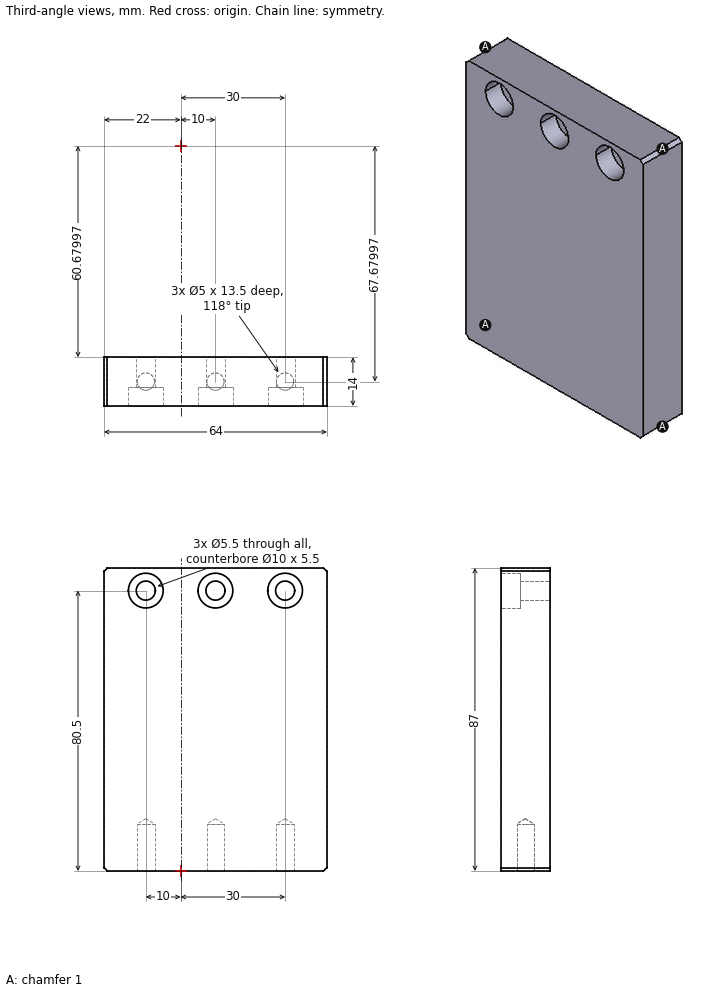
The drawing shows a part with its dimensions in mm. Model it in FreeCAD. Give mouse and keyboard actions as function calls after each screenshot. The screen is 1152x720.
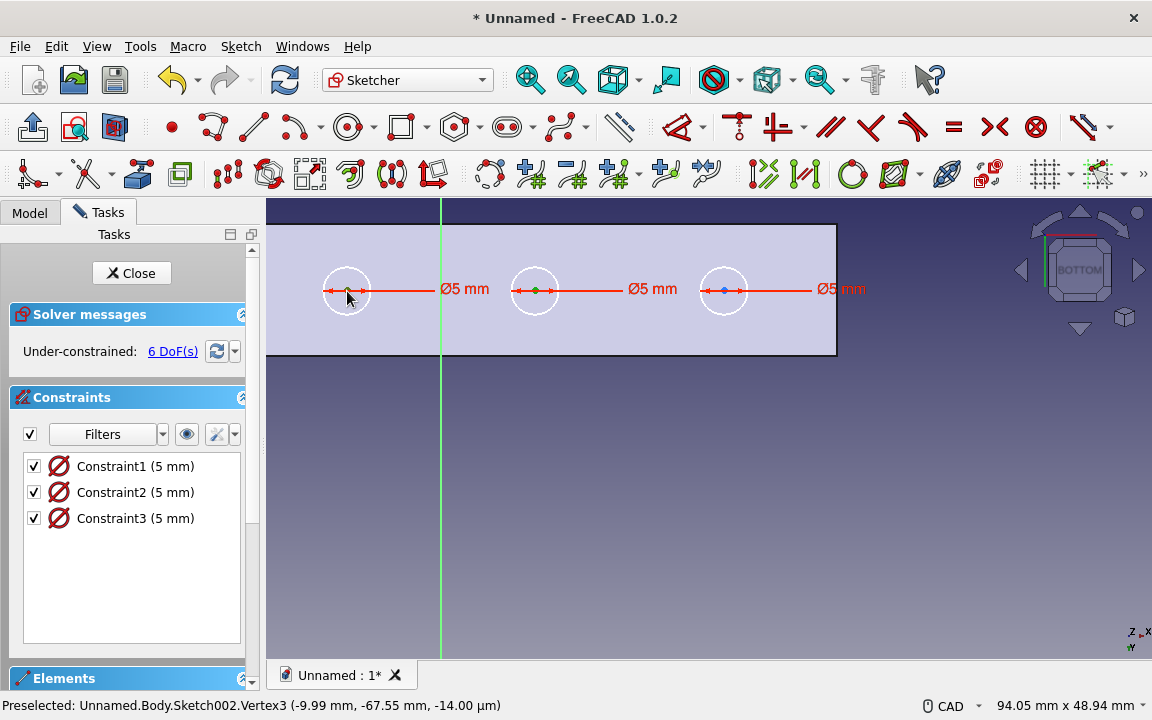
click(441, 602)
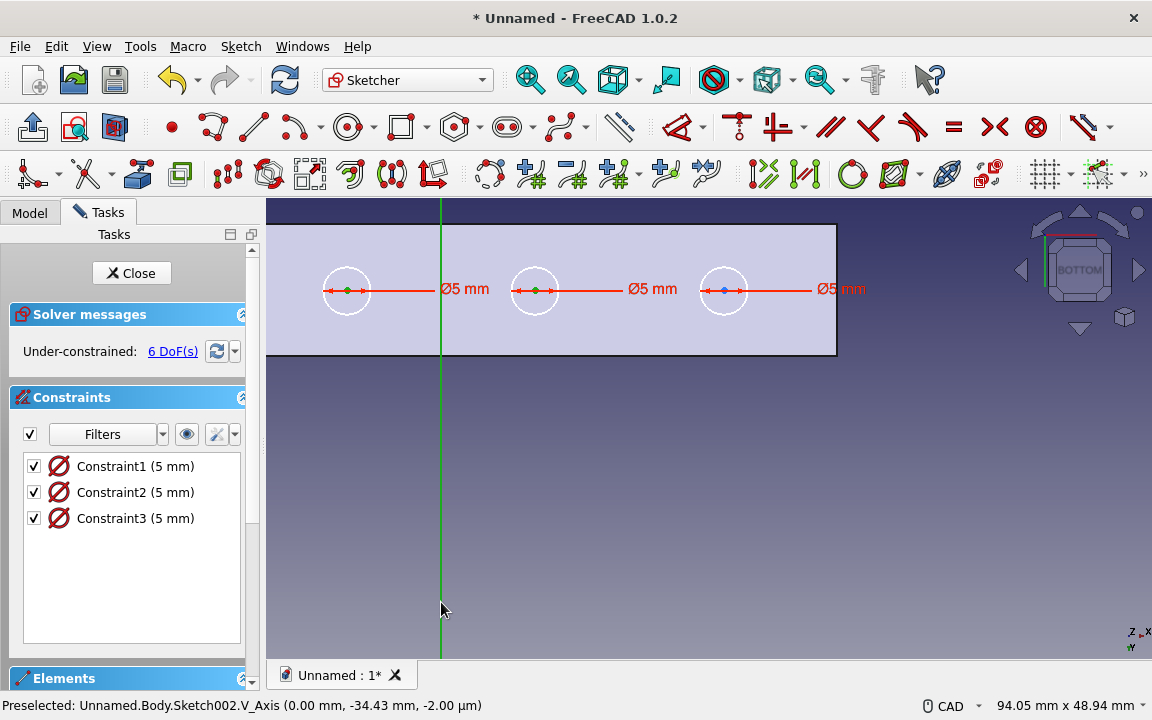
key(s)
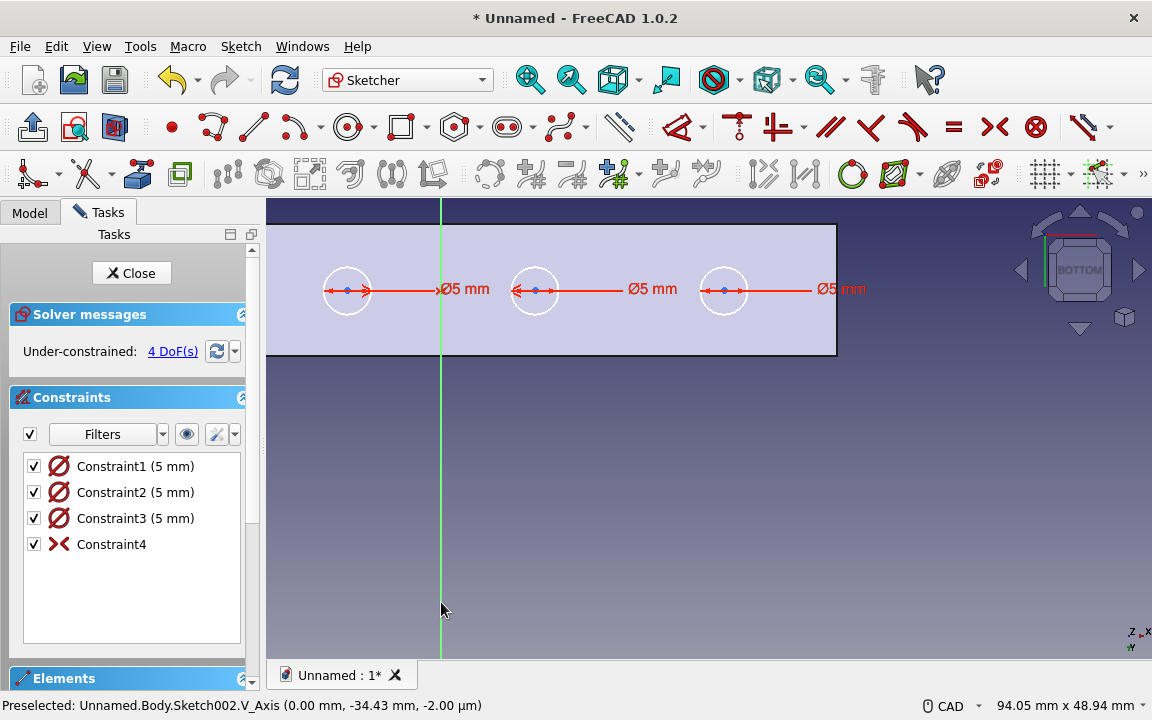
key(d)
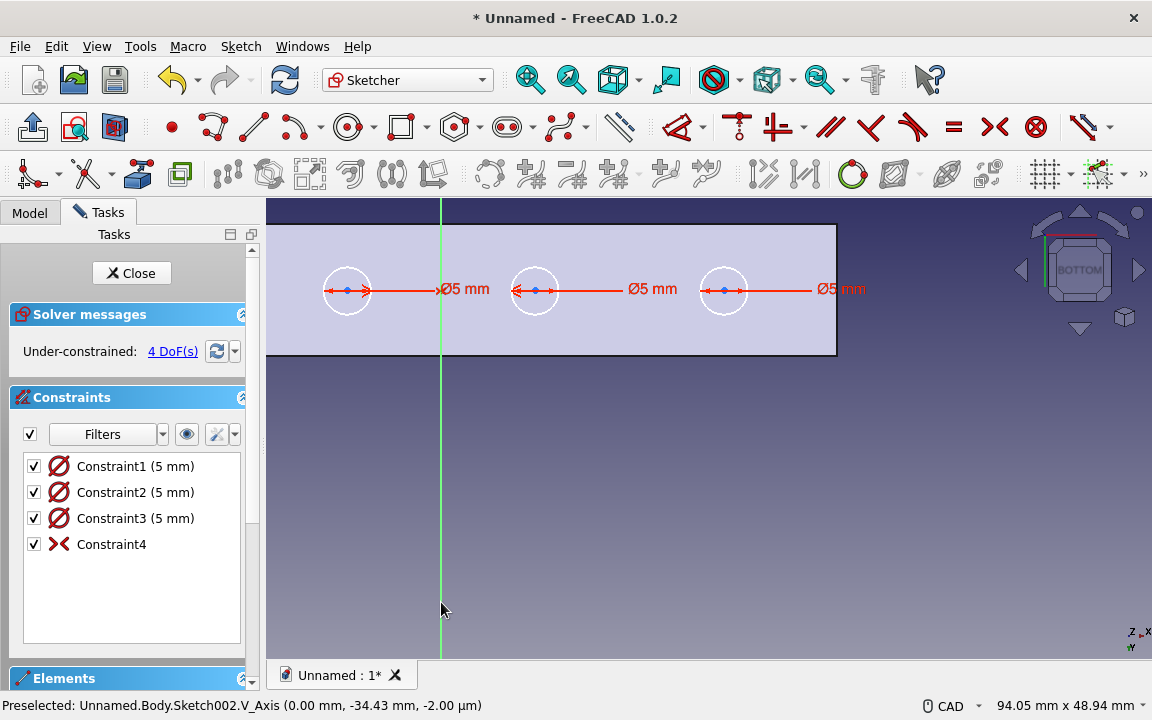
click(724, 291)
click(583, 257)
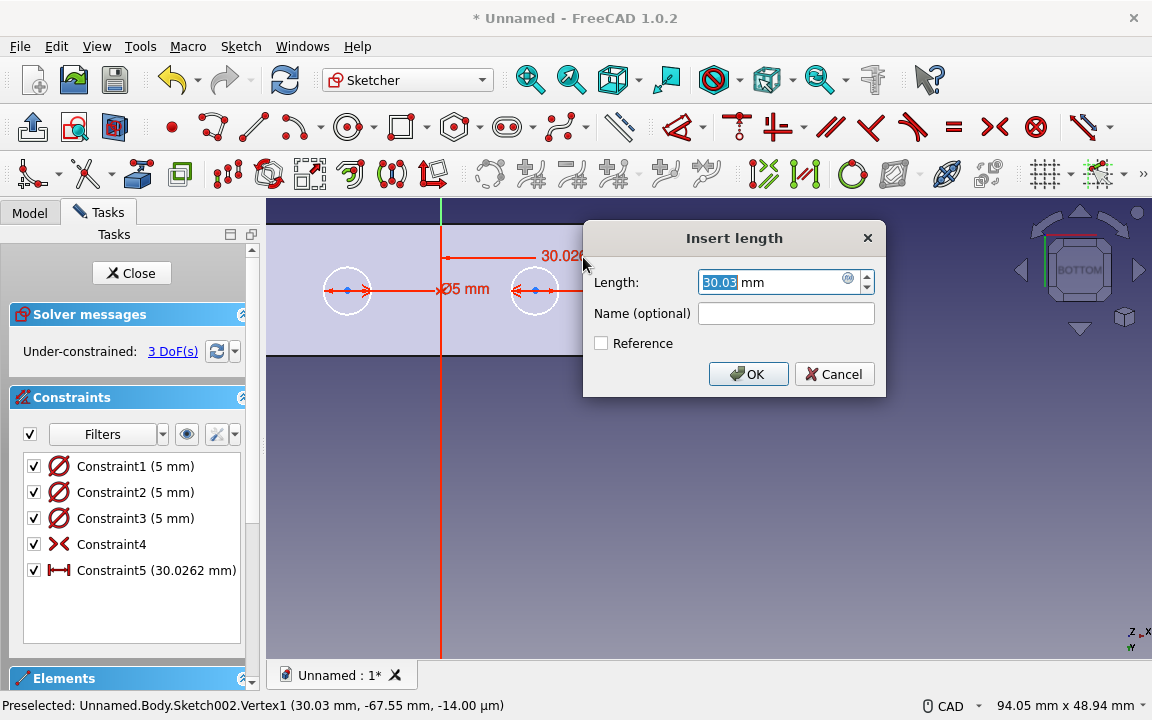
text(30)
key(Return)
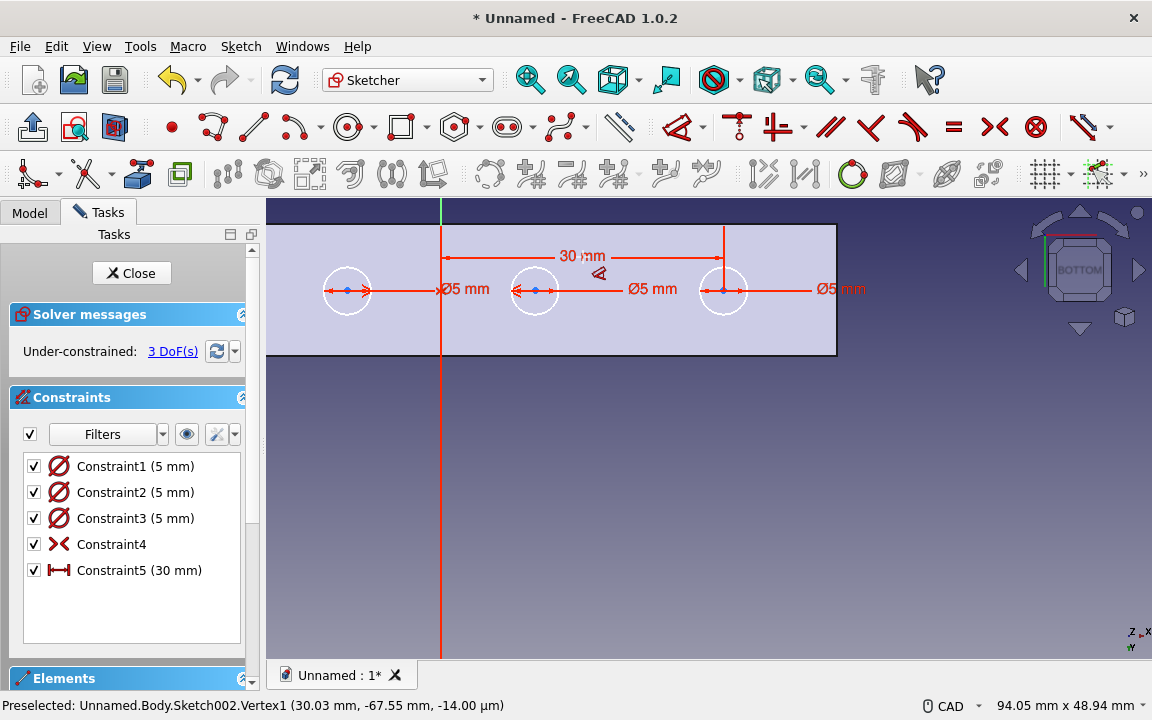
click(535, 291)
click(488, 257)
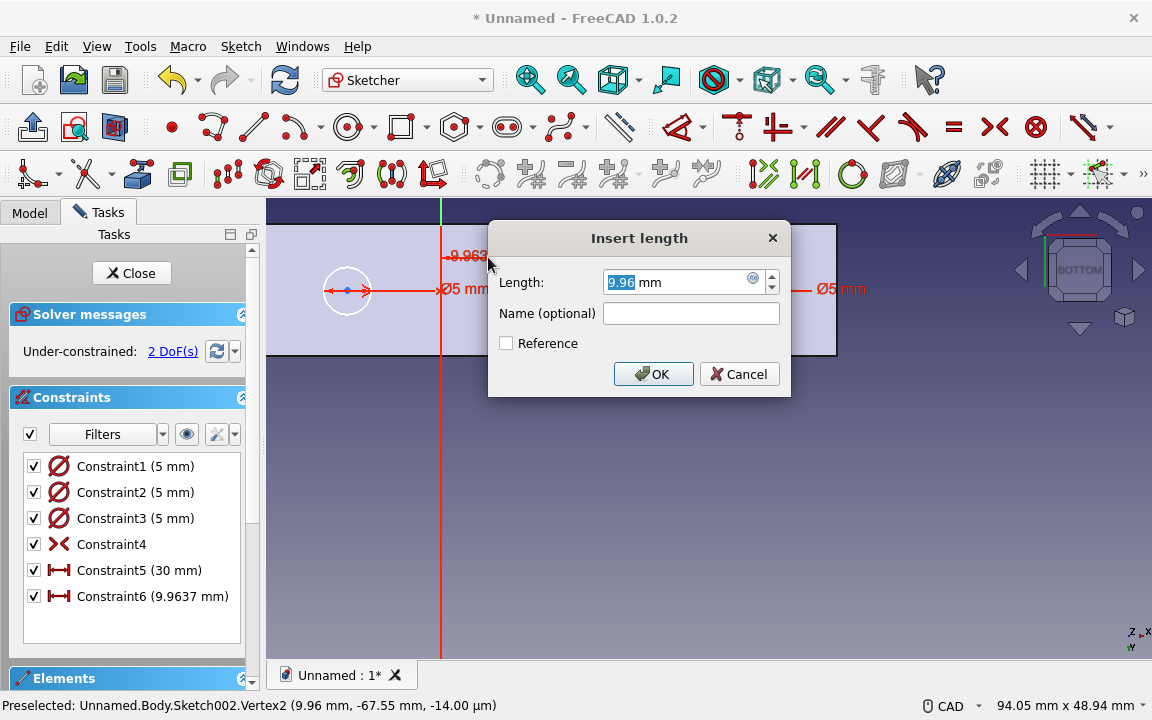
text(10)
key(Return)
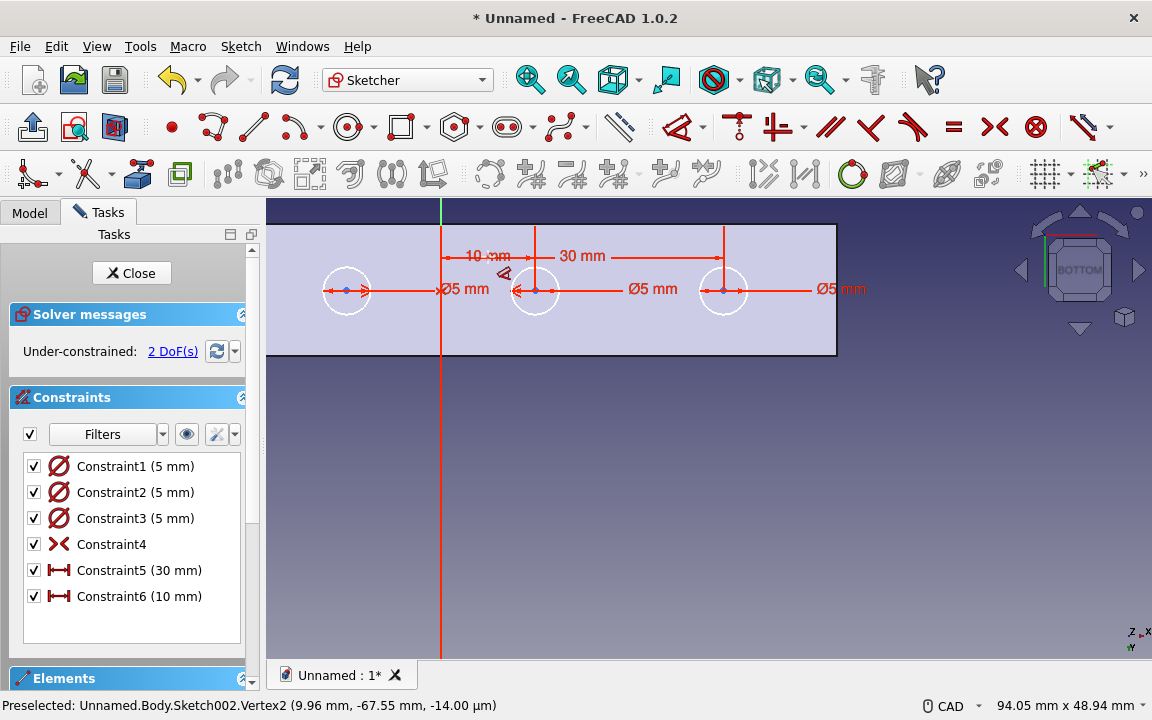
click(724, 291)
click(758, 461)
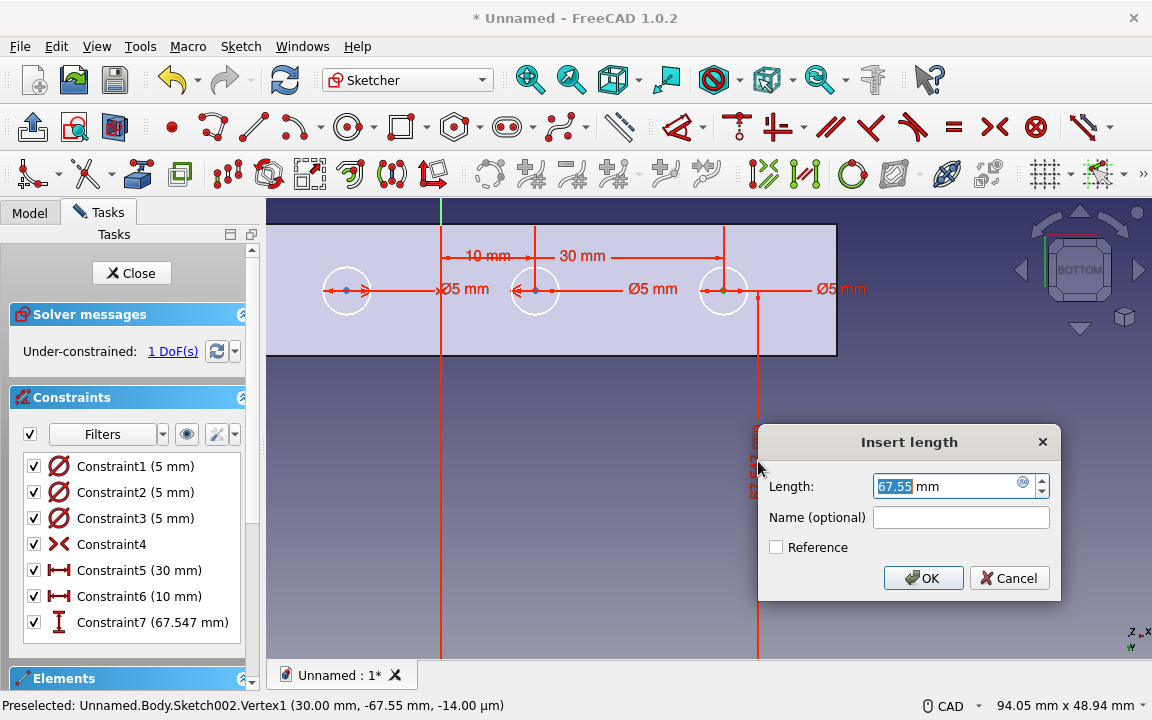
text(67.67997)
key(Return)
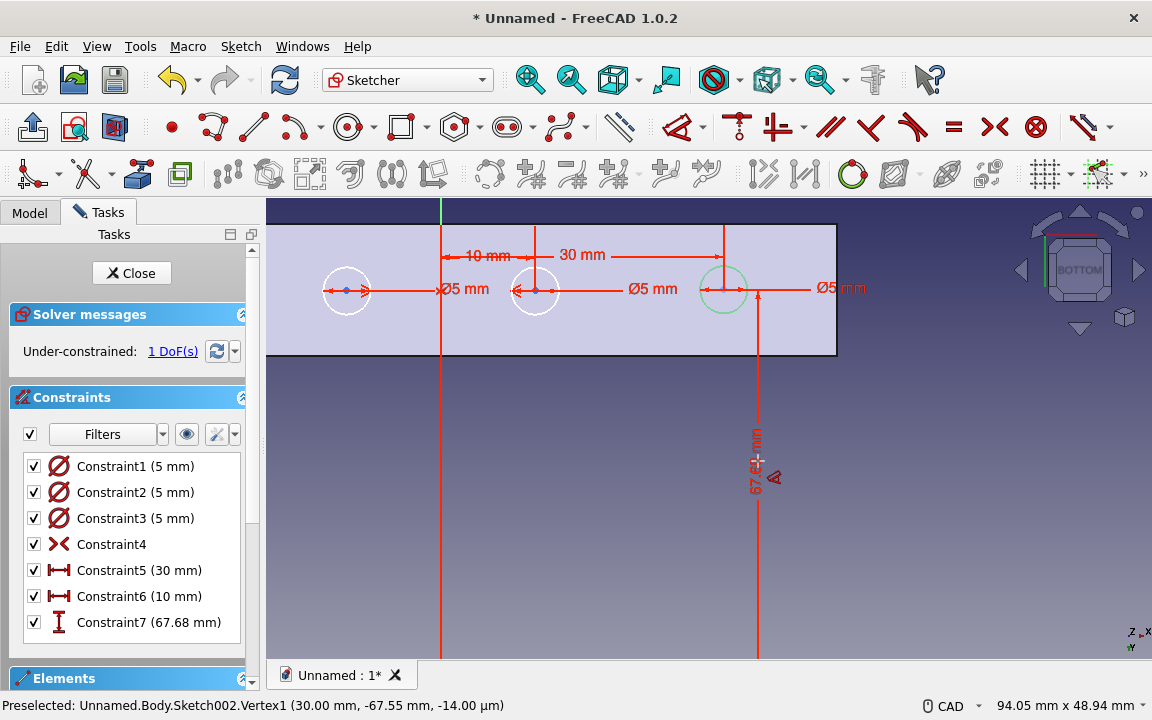
click(535, 291)
click(407, 461)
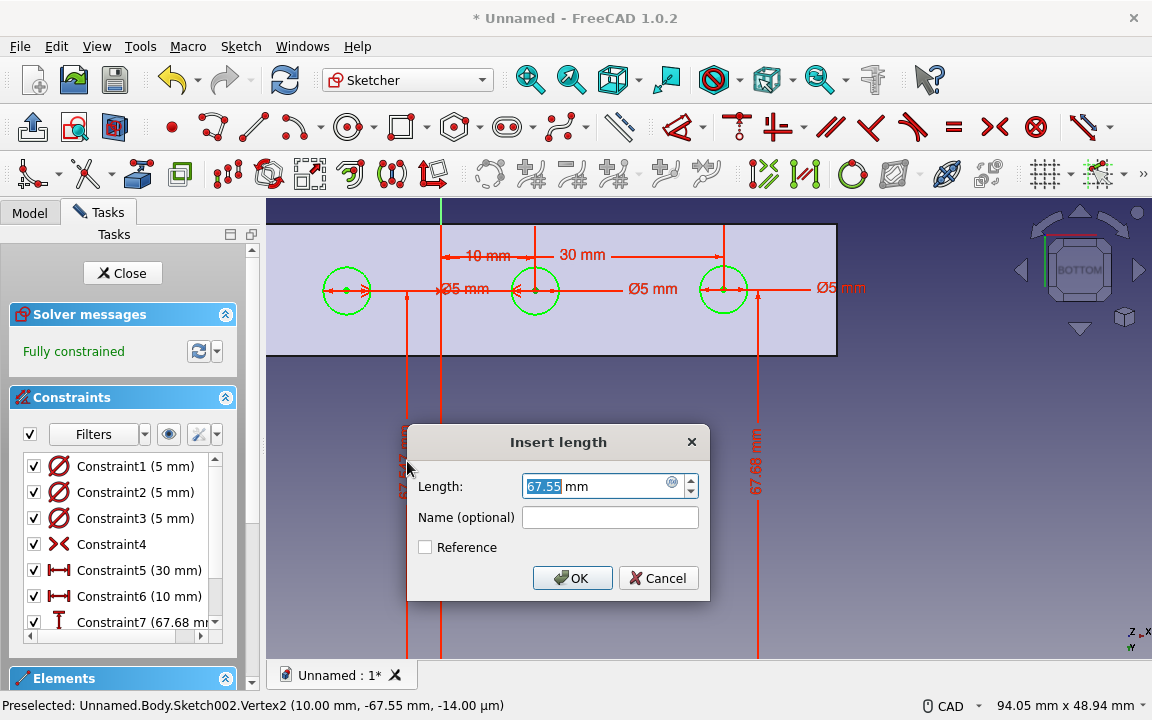
text(67.67997)
key(Return)
key(Escape)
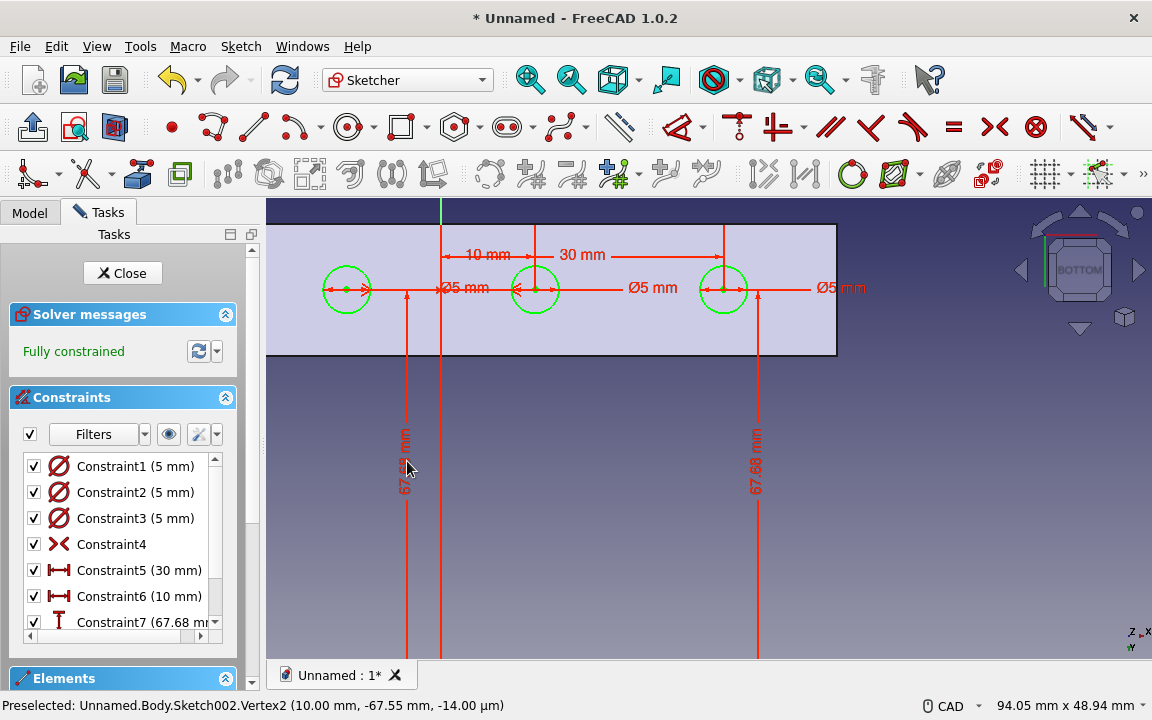
click(123, 273)